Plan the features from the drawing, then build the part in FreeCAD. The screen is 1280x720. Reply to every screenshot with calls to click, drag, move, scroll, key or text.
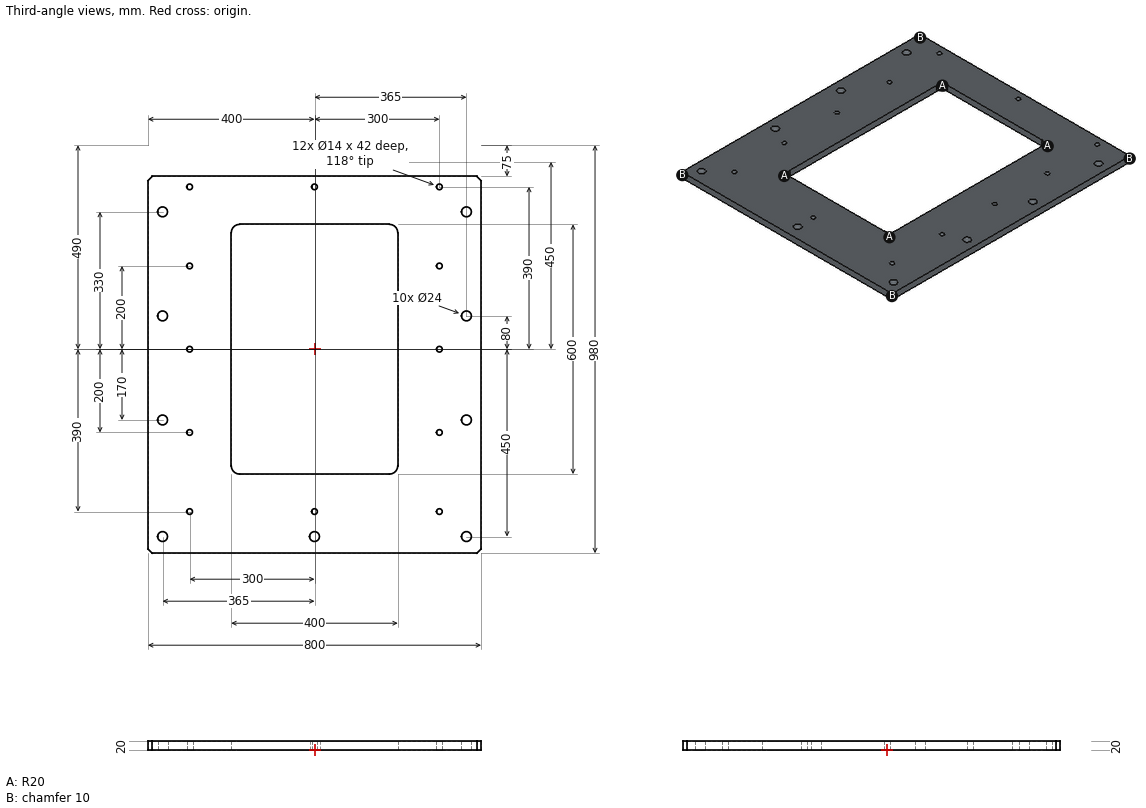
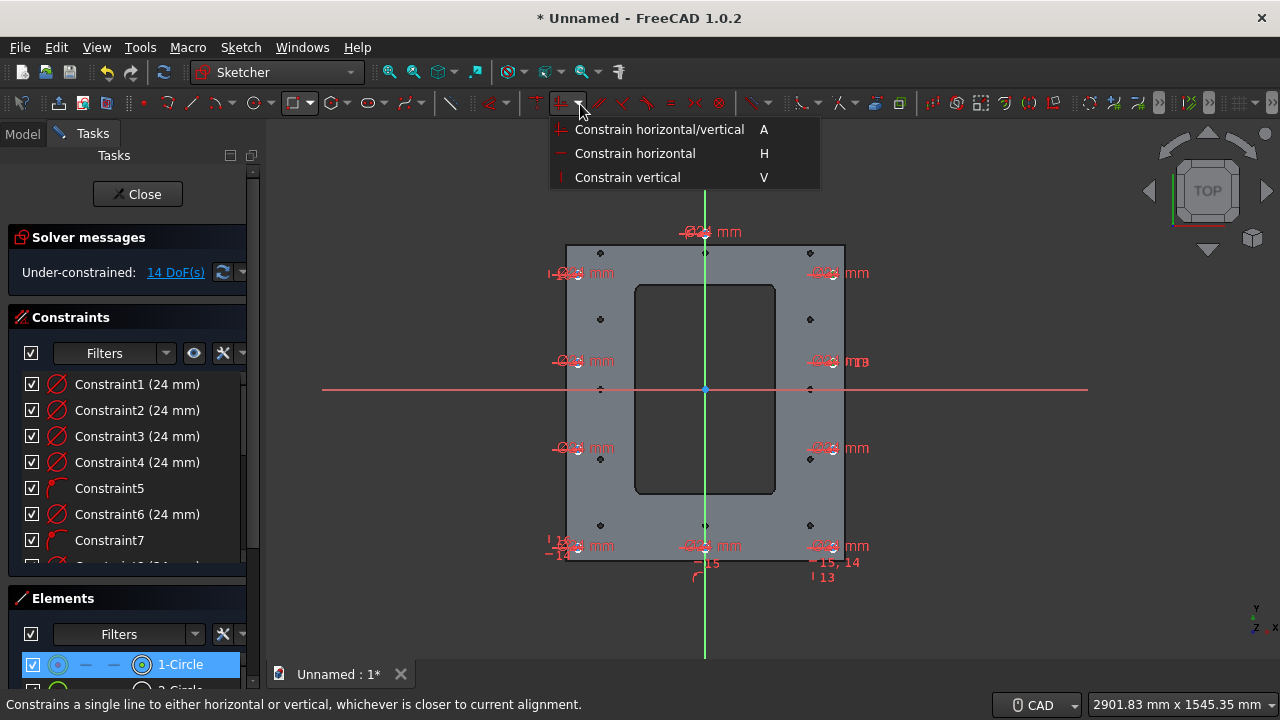
click(685, 177)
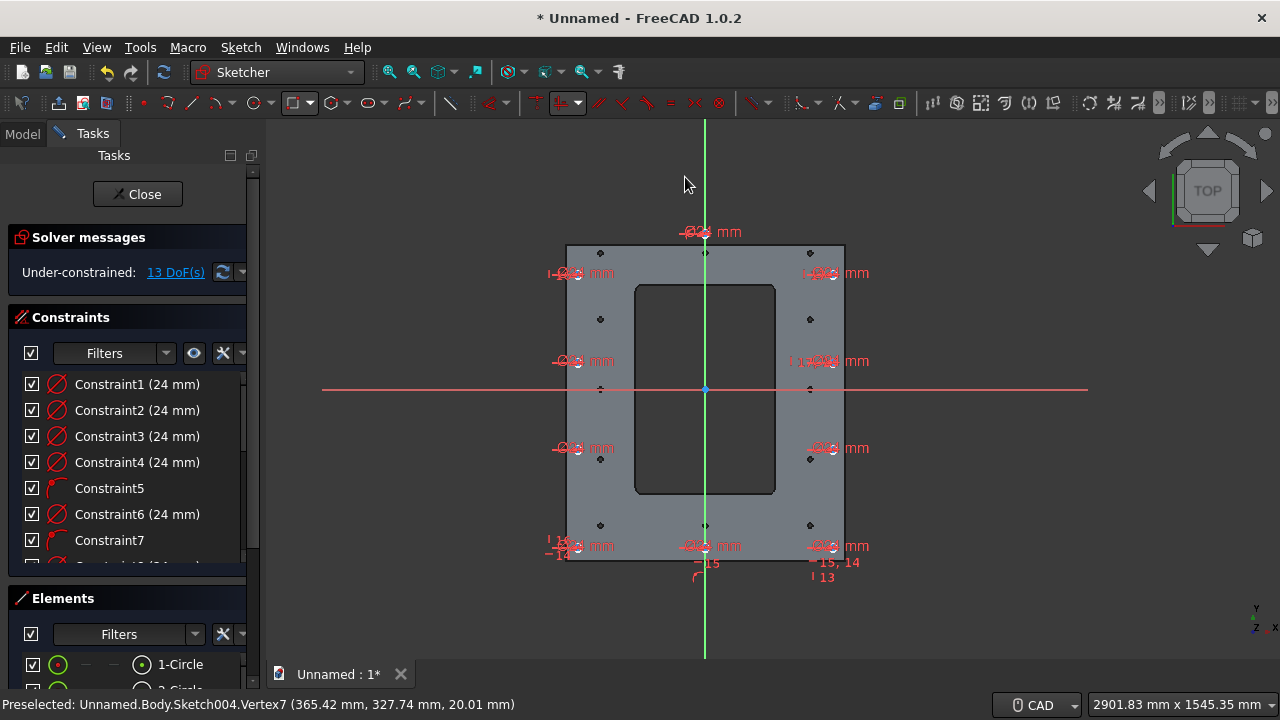
click(578, 275)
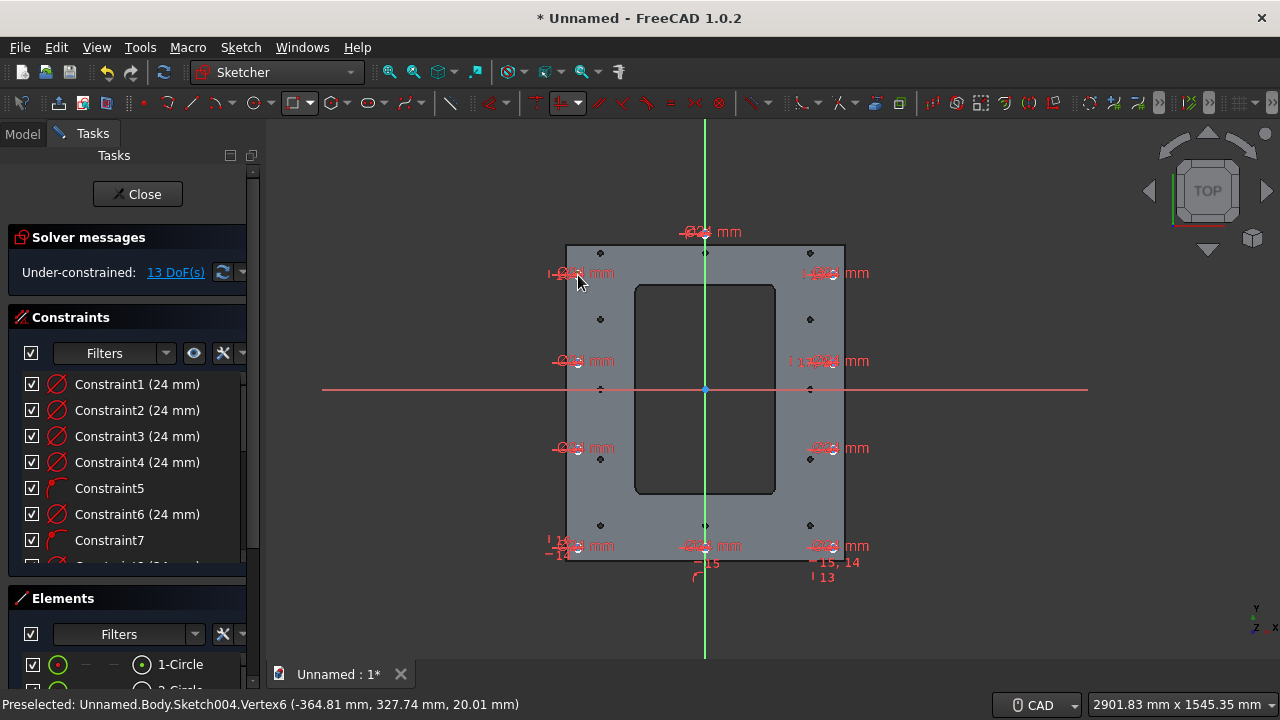
click(833, 275)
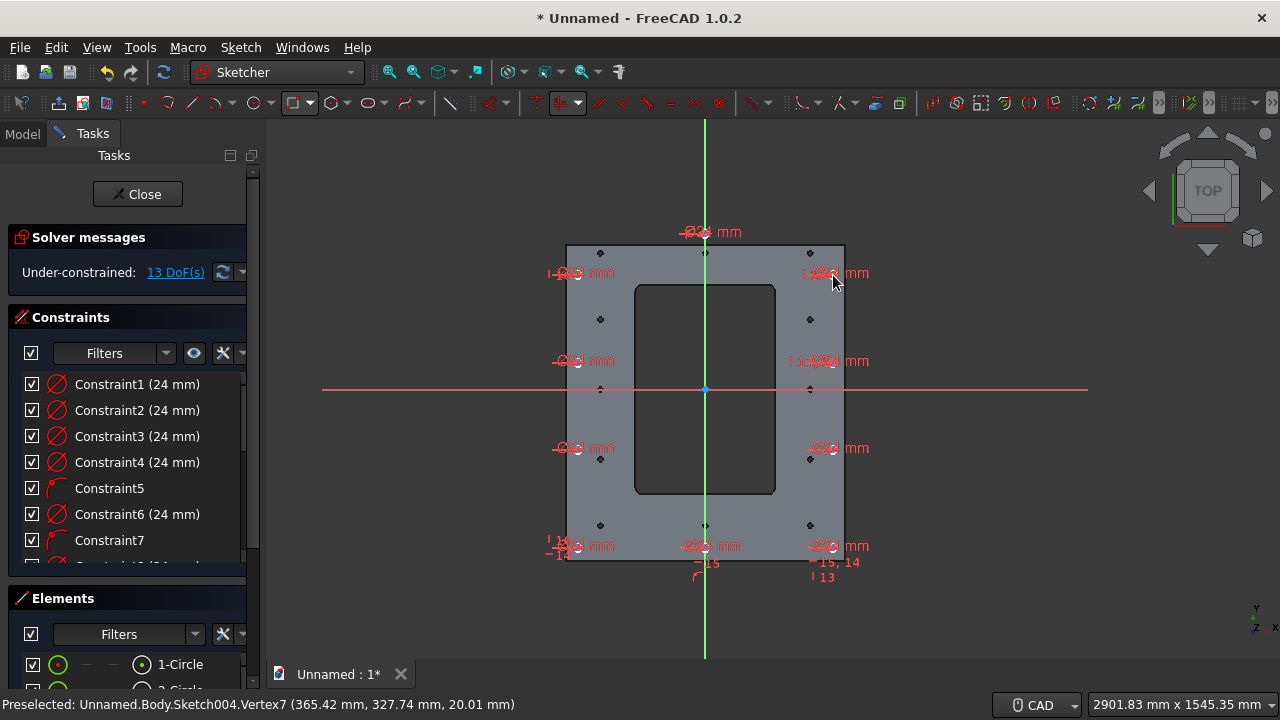
key(h)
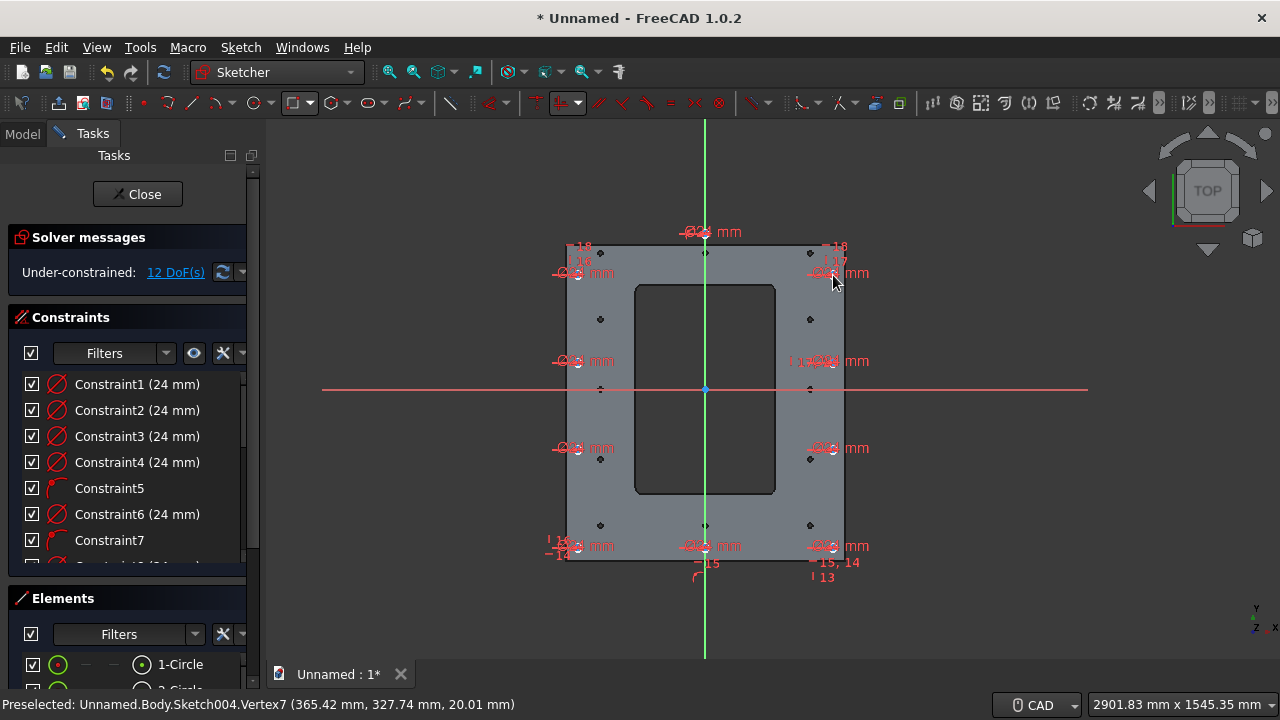
click(578, 275)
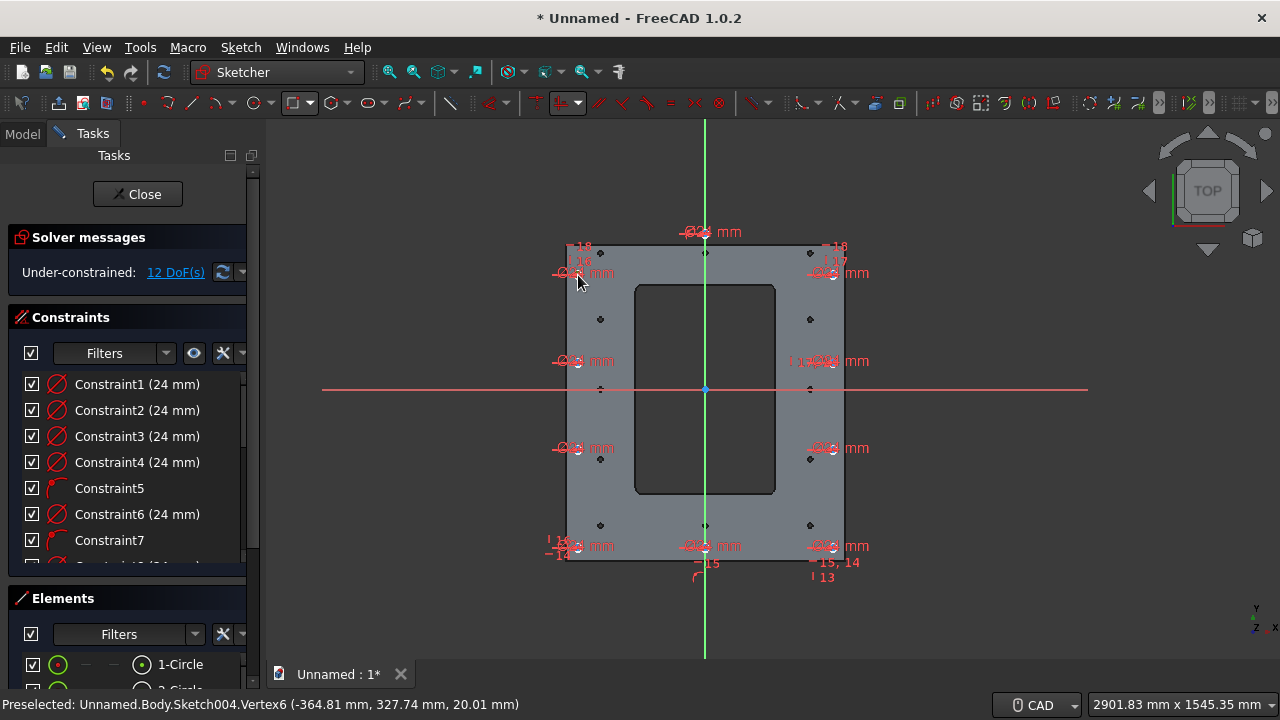
click(578, 363)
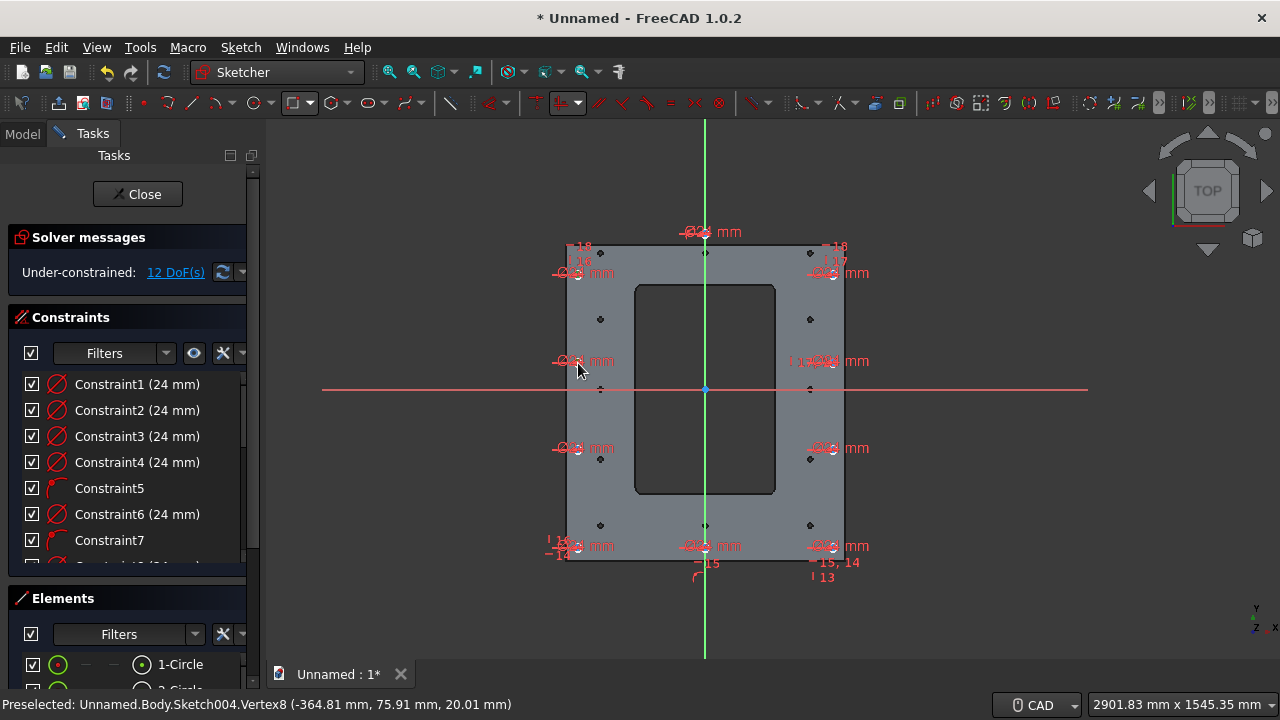
click(580, 104)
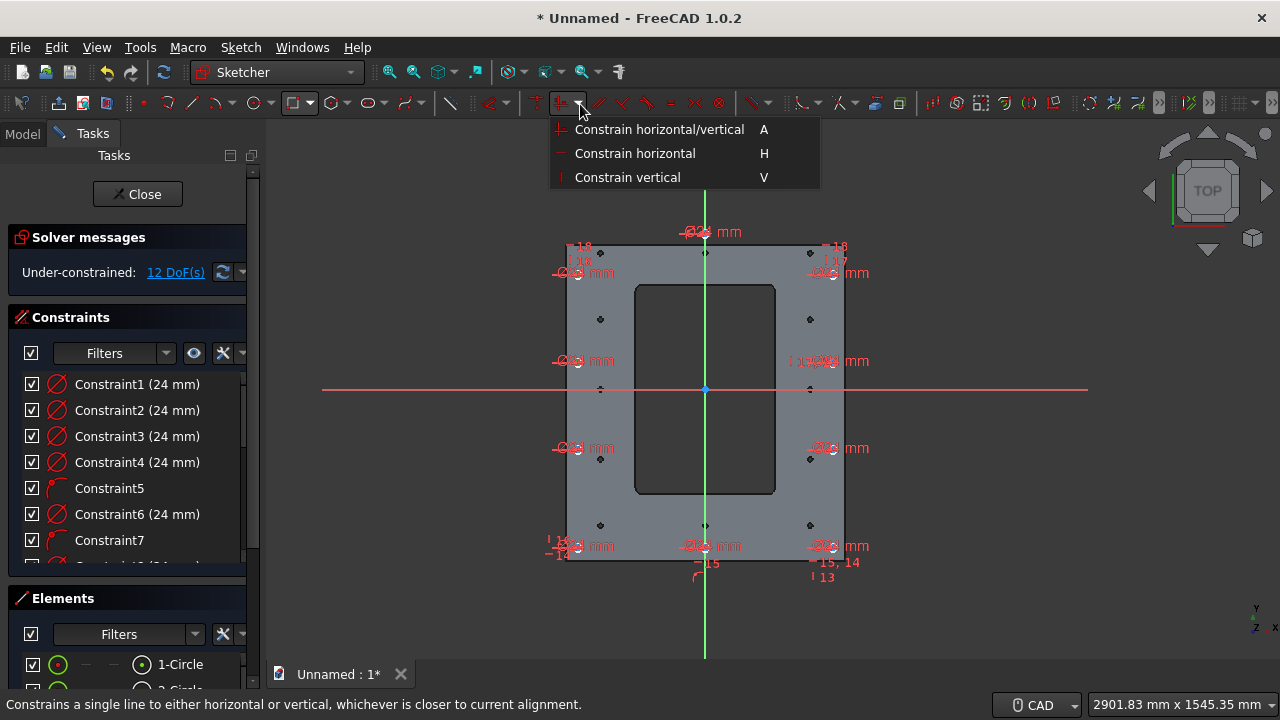
click(685, 177)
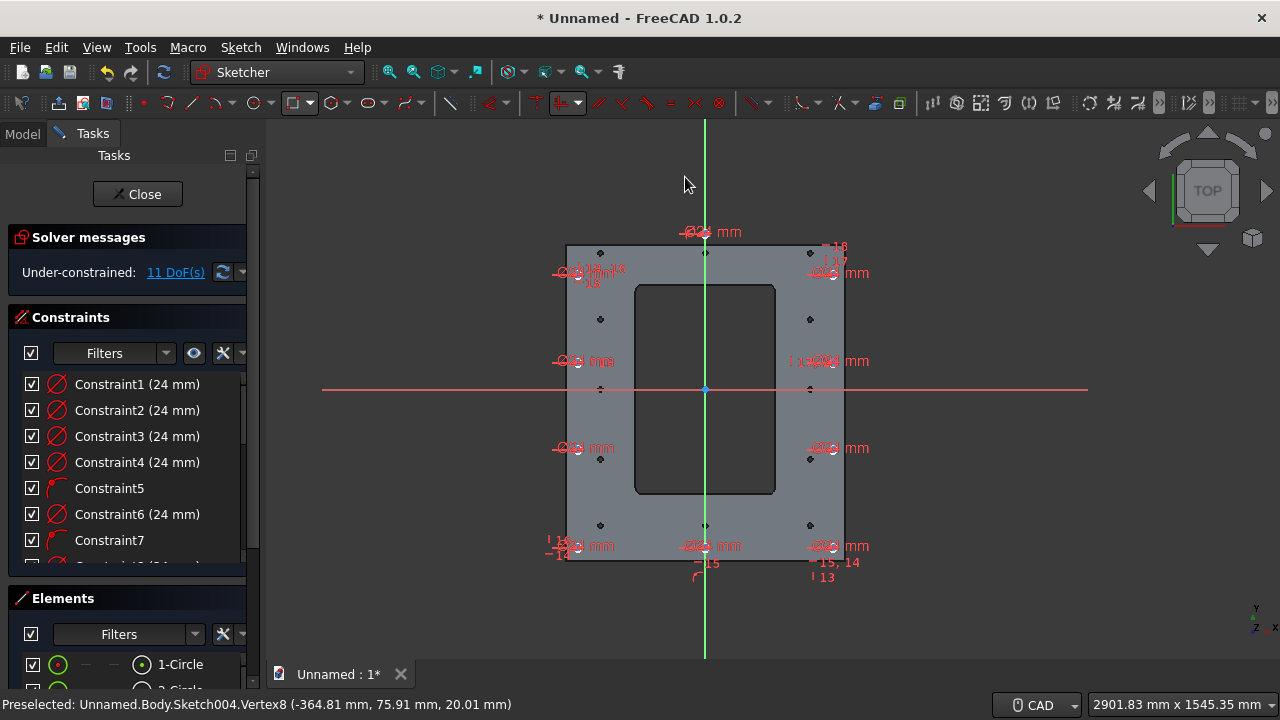
click(833, 363)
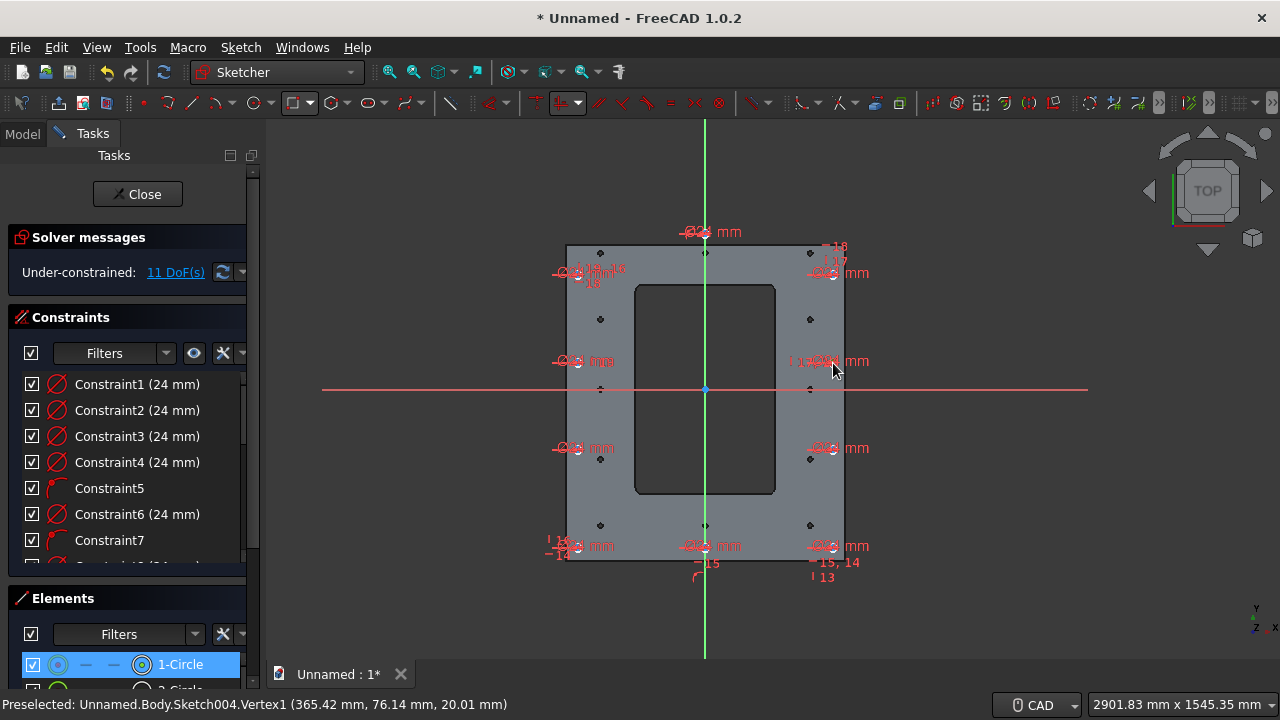
click(578, 363)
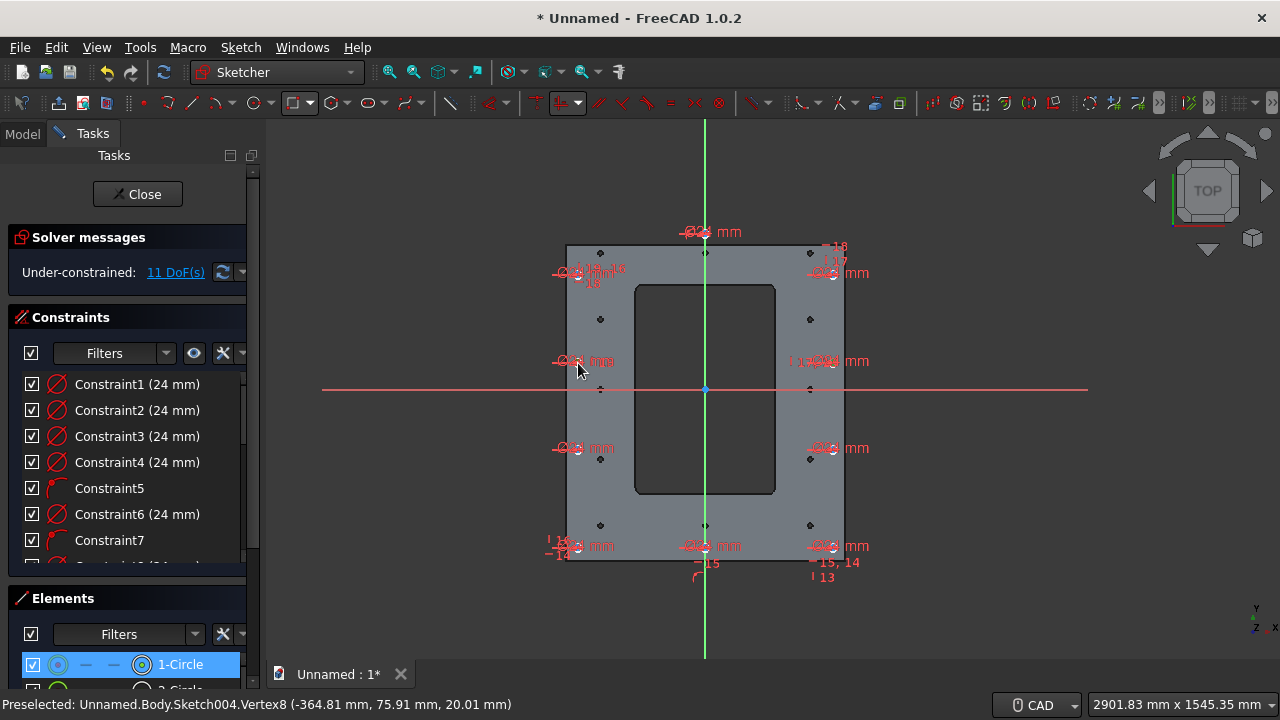
key(h)